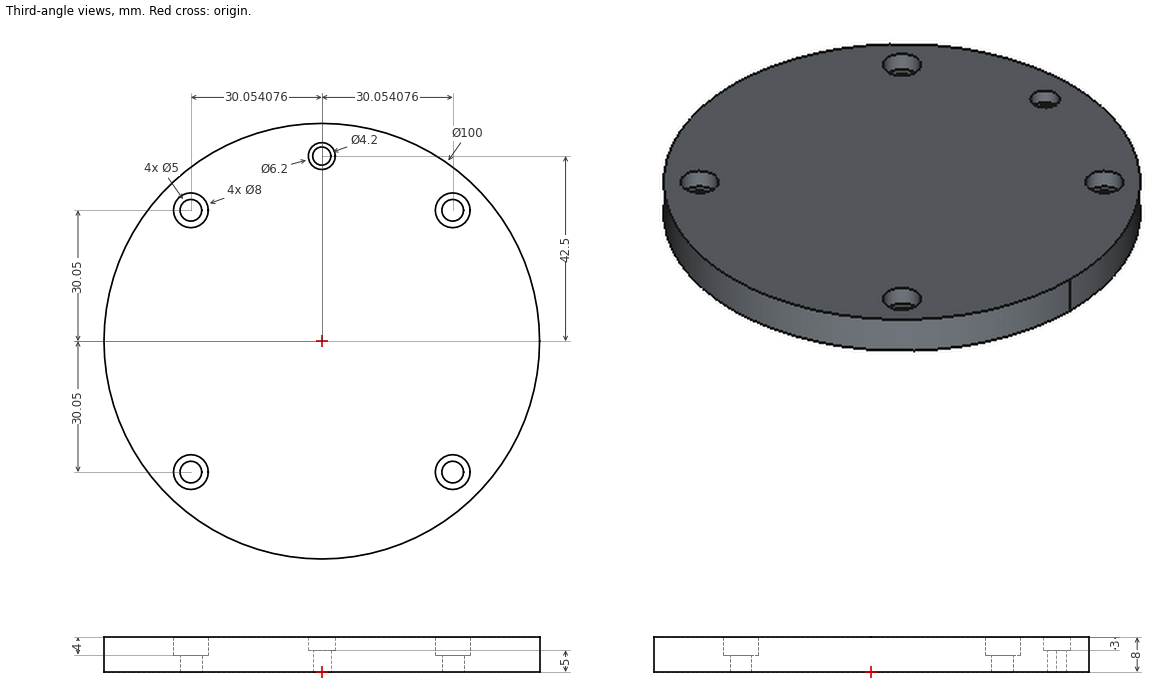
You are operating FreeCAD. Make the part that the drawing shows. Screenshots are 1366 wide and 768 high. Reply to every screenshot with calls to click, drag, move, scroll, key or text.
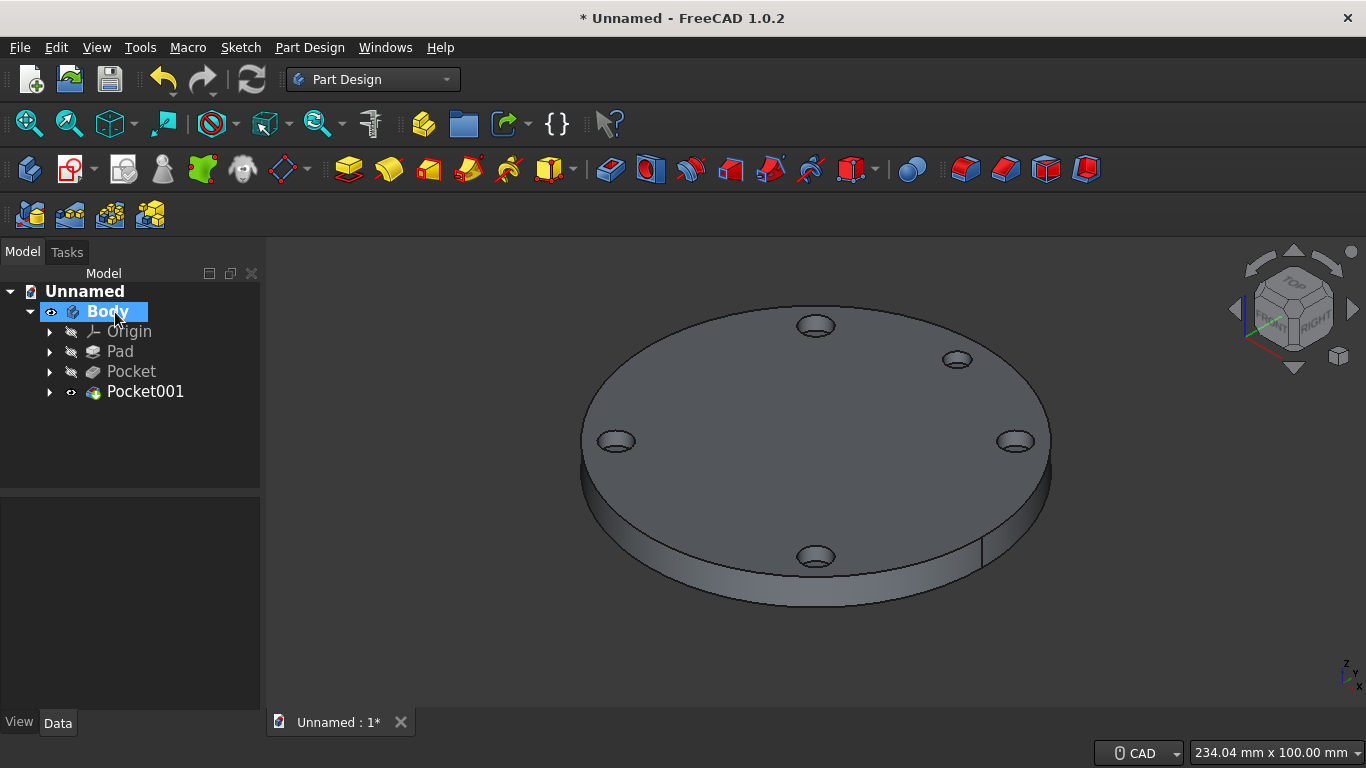
key(2)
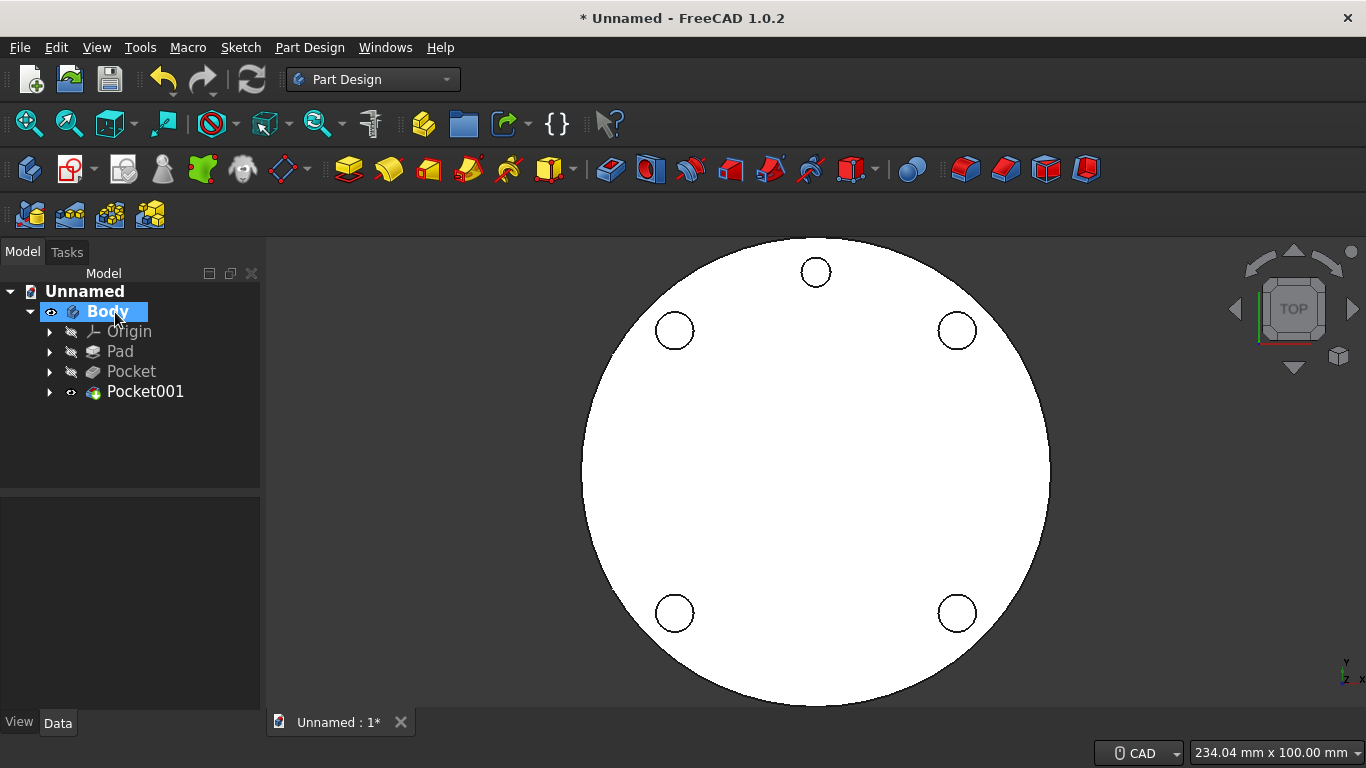
click(30, 124)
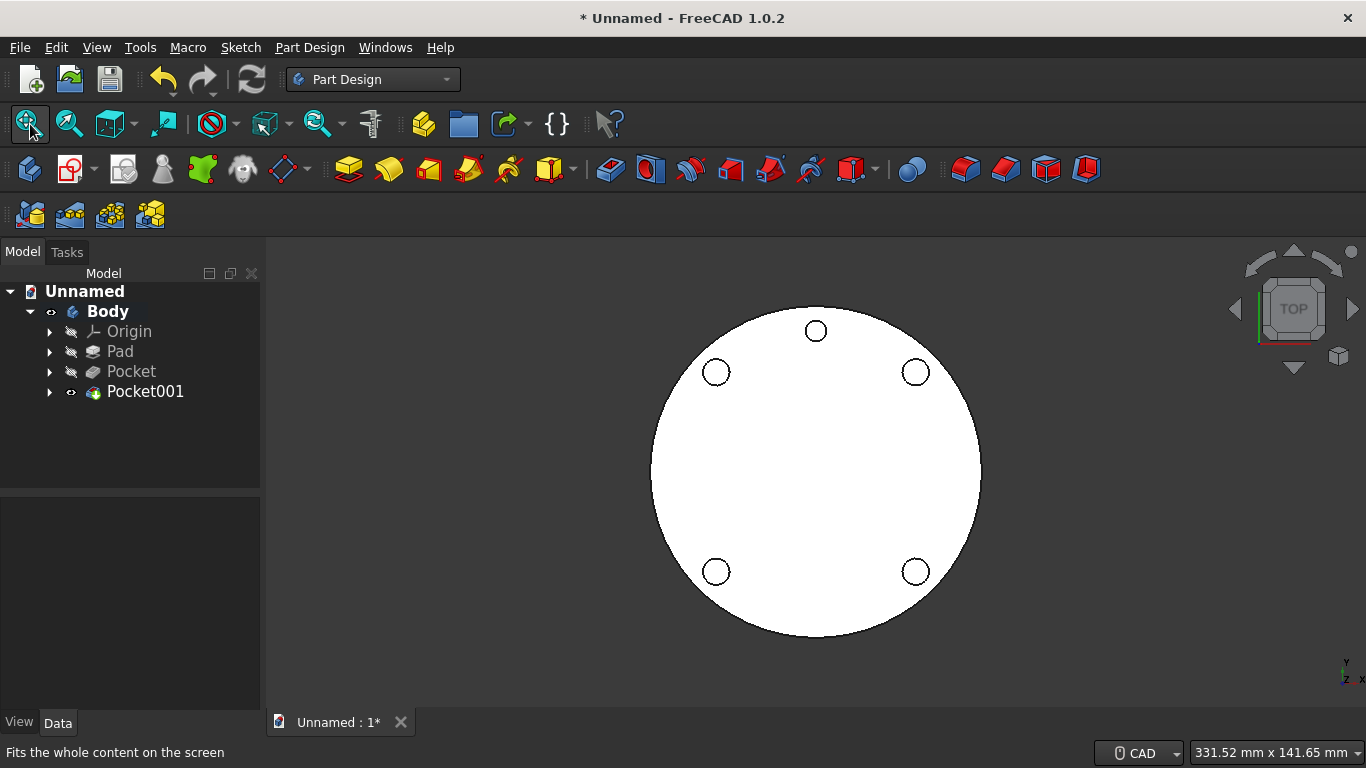
click(716, 571)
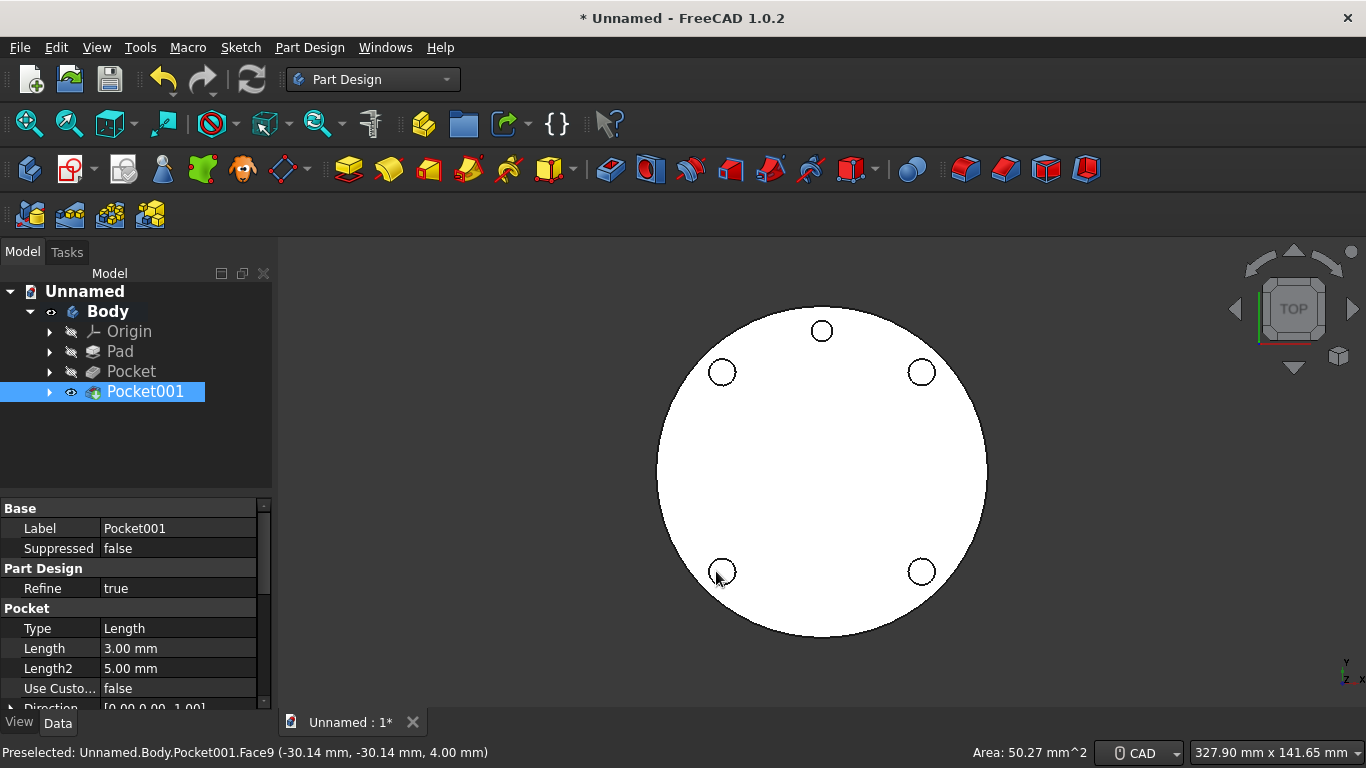
click(70, 170)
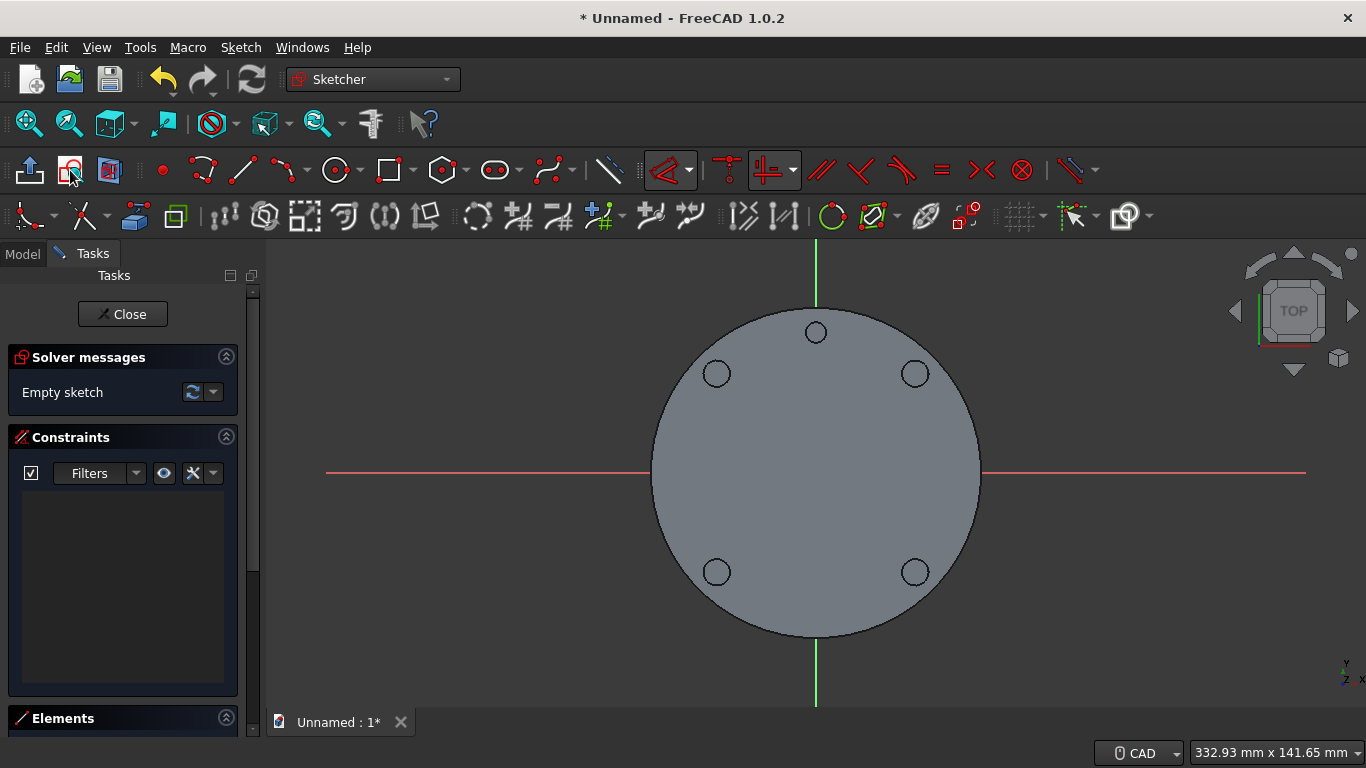
click(336, 170)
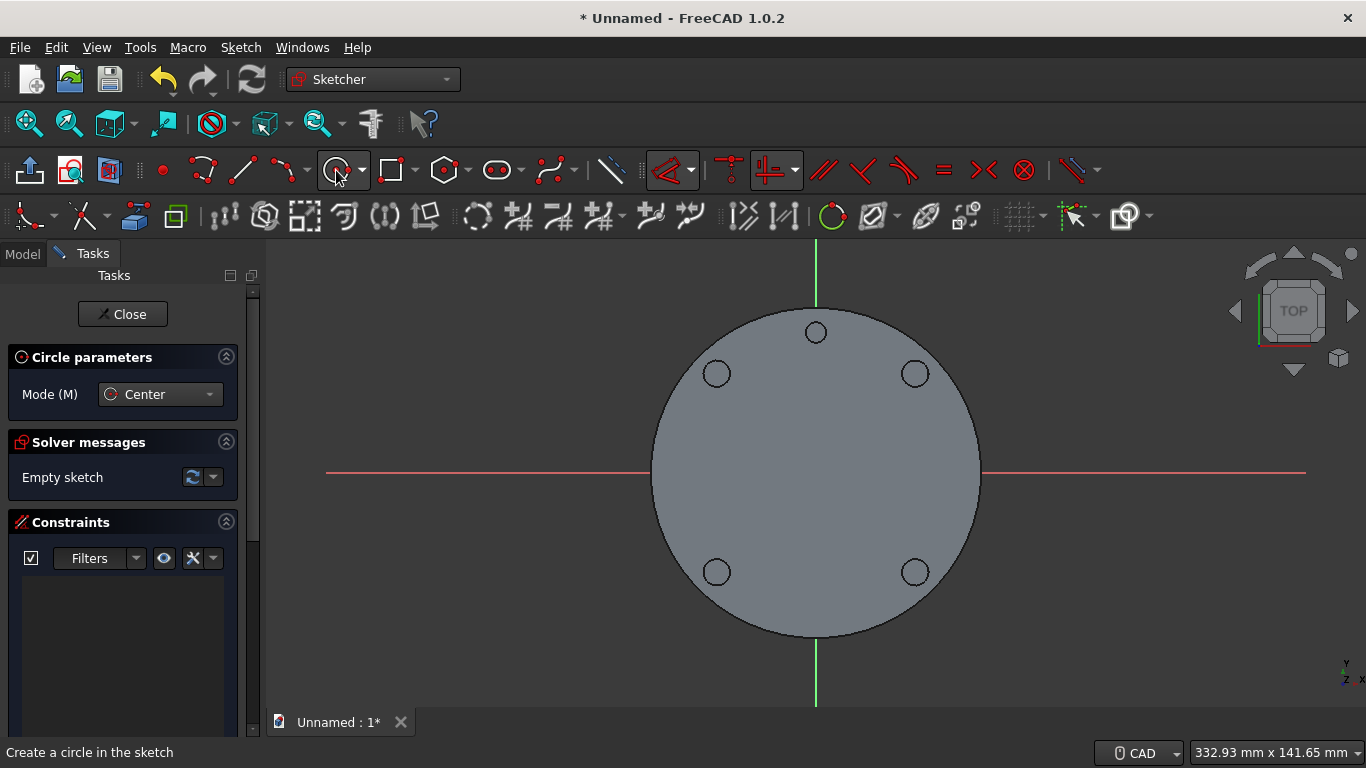
scroll(717, 374, up, 6)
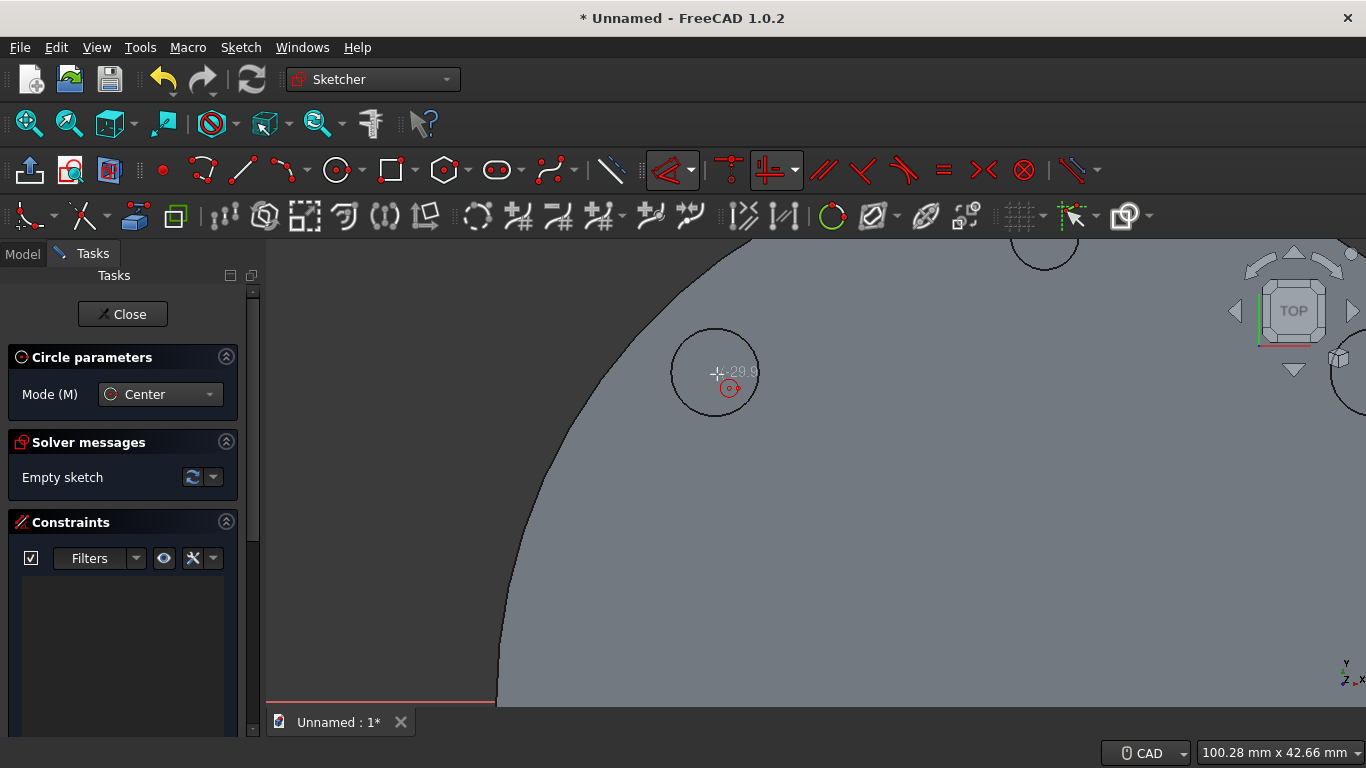
click(715, 372)
move(734, 353)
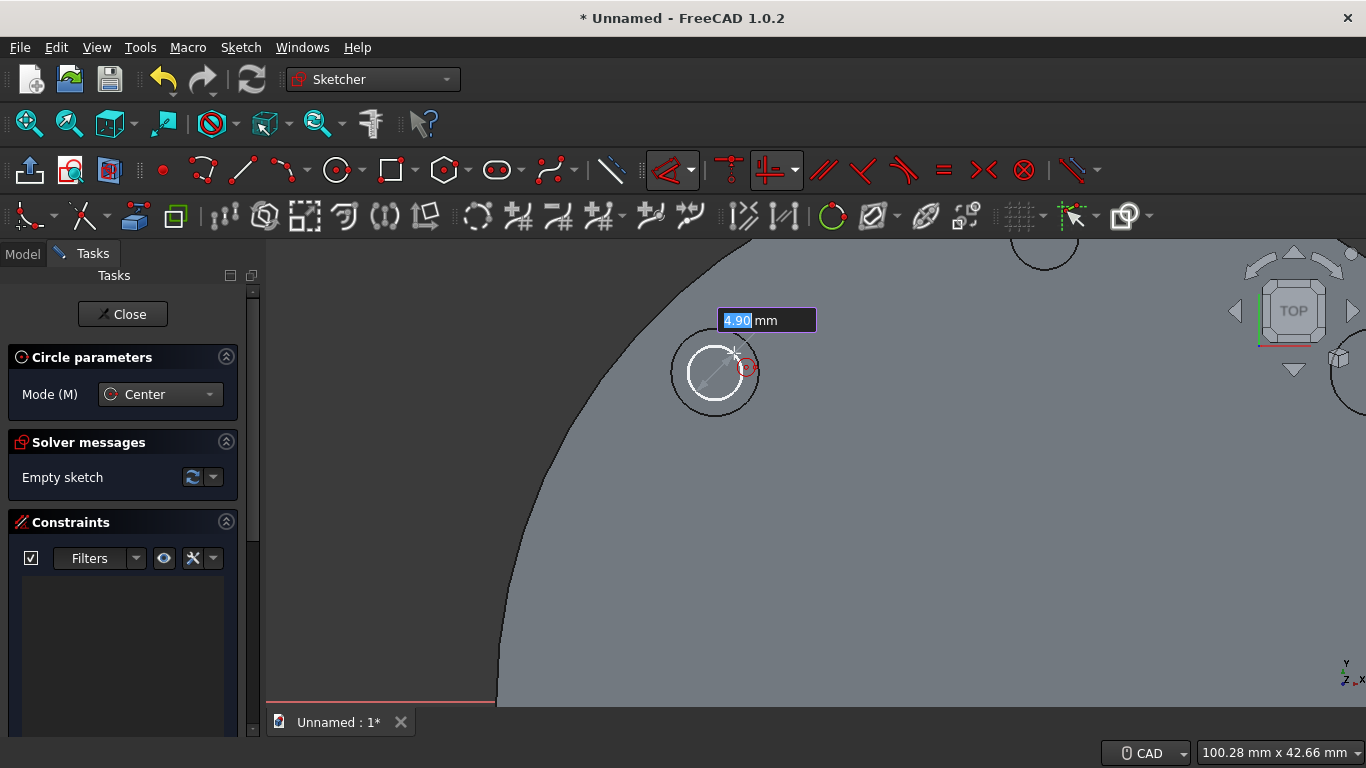
text(5)
key(Return)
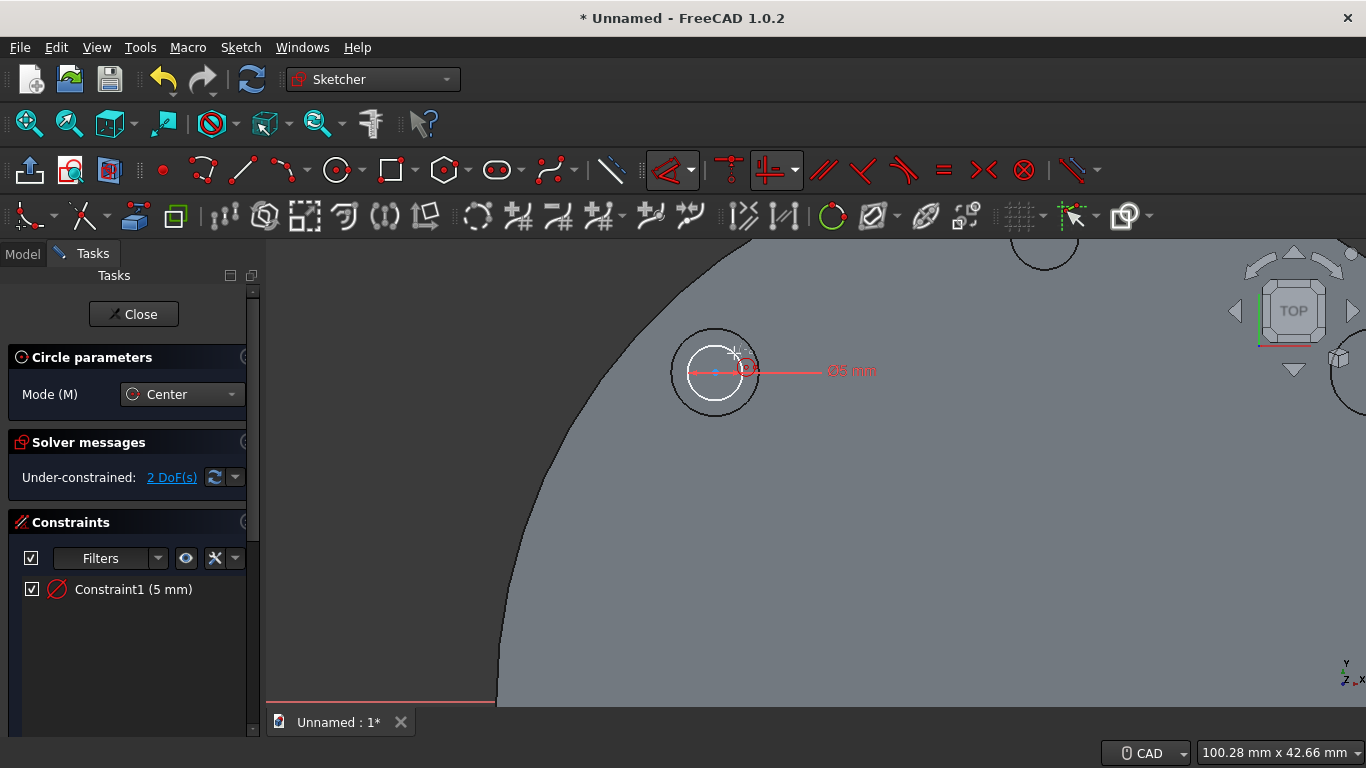
scroll(575, 378, down, 5)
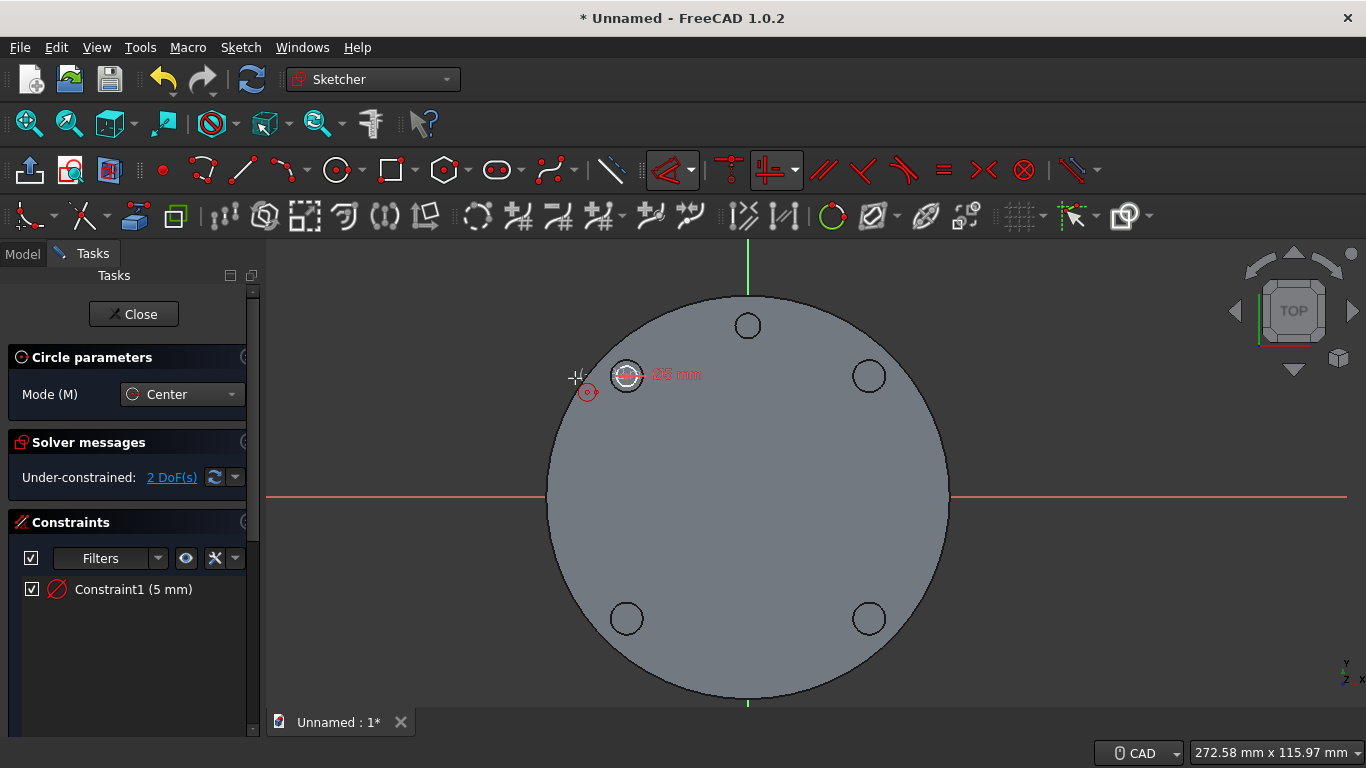
scroll(869, 376, up, 5)